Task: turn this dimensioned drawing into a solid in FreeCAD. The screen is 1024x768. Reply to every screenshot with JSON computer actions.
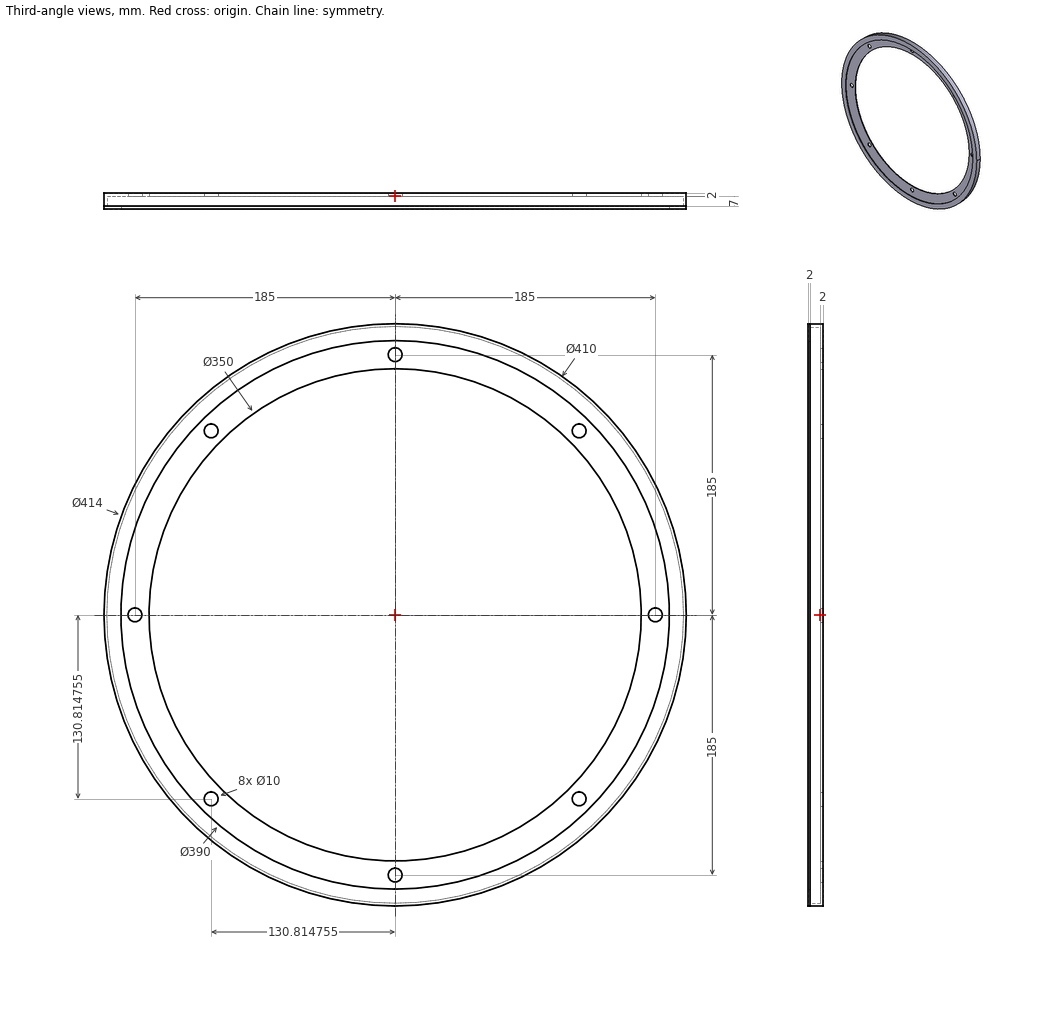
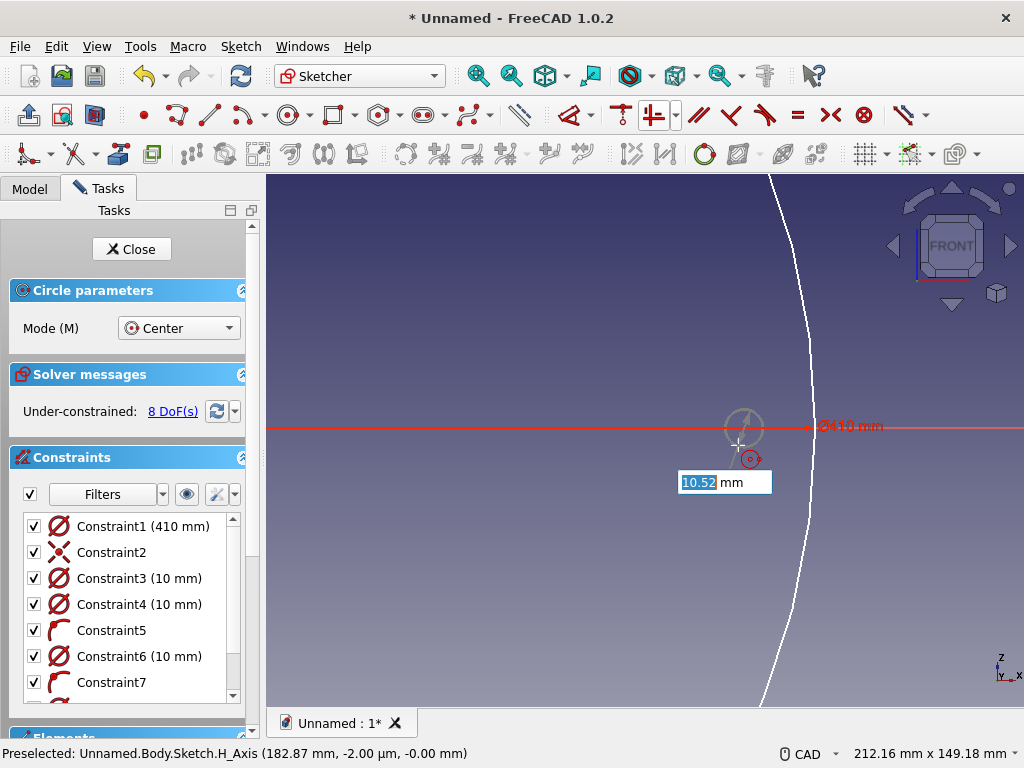
{"action": "type", "text": "10"}
{"action": "key", "text": "Return"}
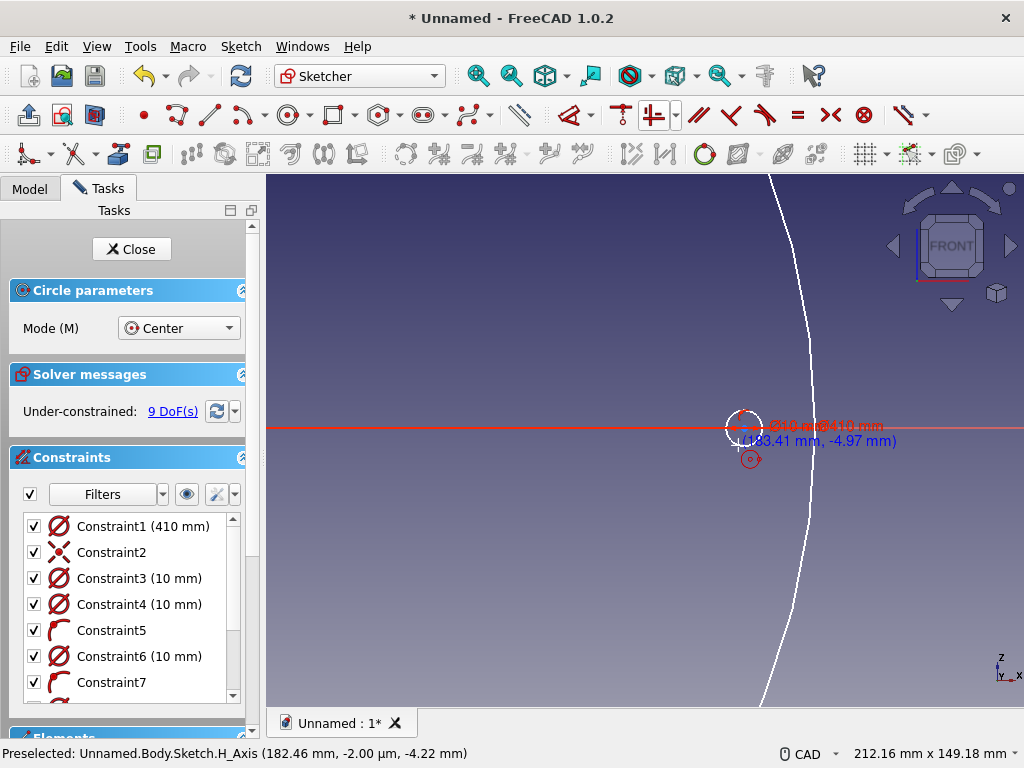
{"action": "scroll", "coordinate": [738, 445], "scroll_direction": "down", "scroll_amount": 7}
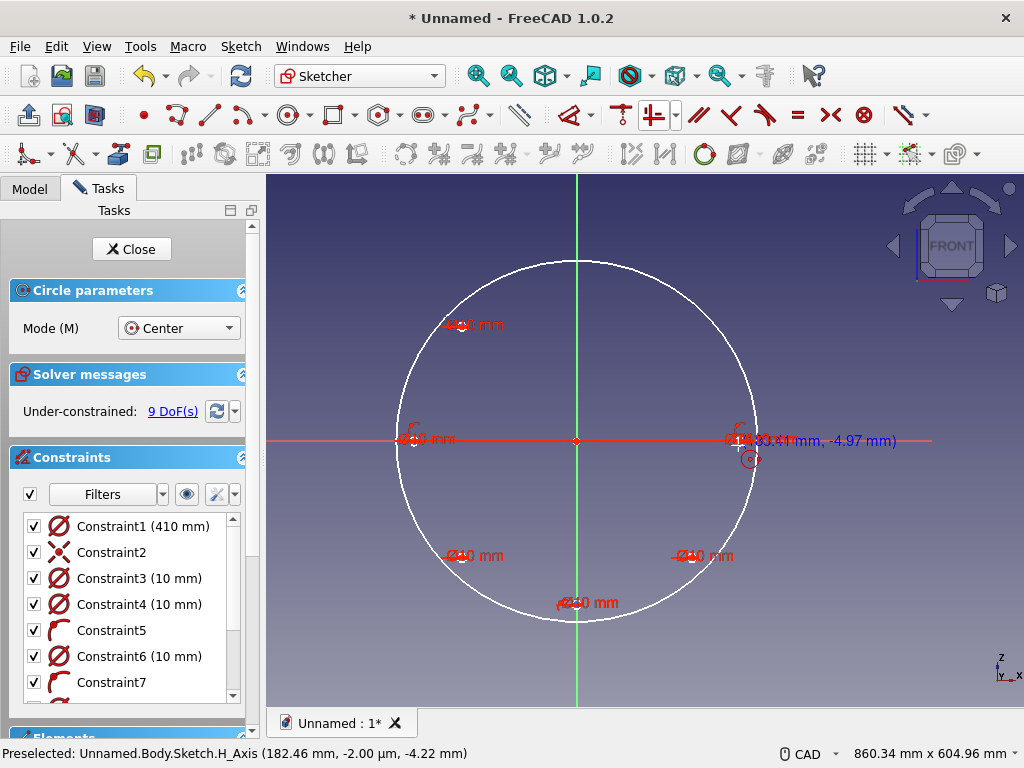
{"action": "left_click", "coordinate": [577, 441]}
{"action": "mouse_move", "coordinate": [686, 332]}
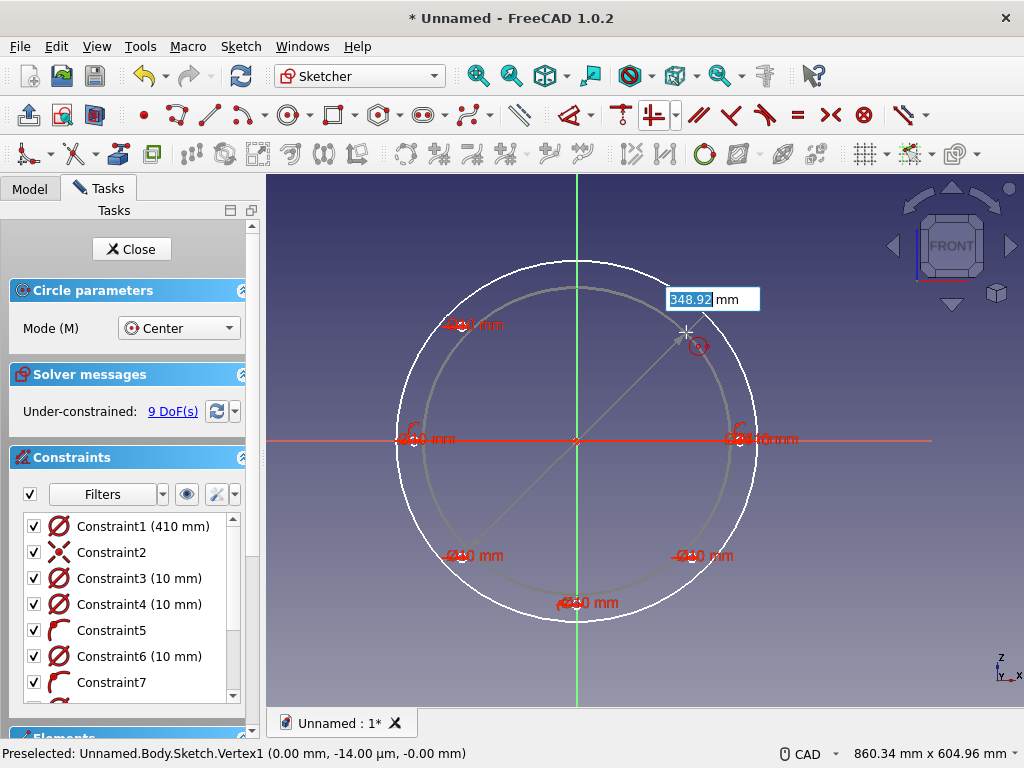
{"action": "type", "text": "350"}
{"action": "key", "text": "Return"}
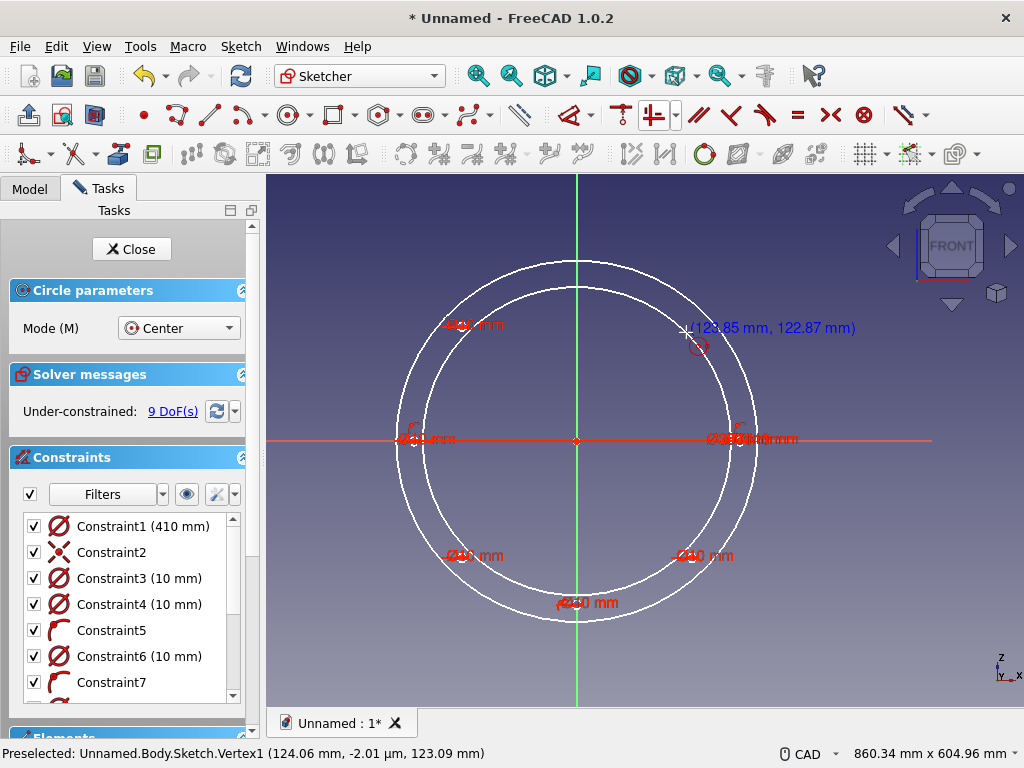
{"action": "scroll", "coordinate": [577, 278], "scroll_direction": "up", "scroll_amount": 9}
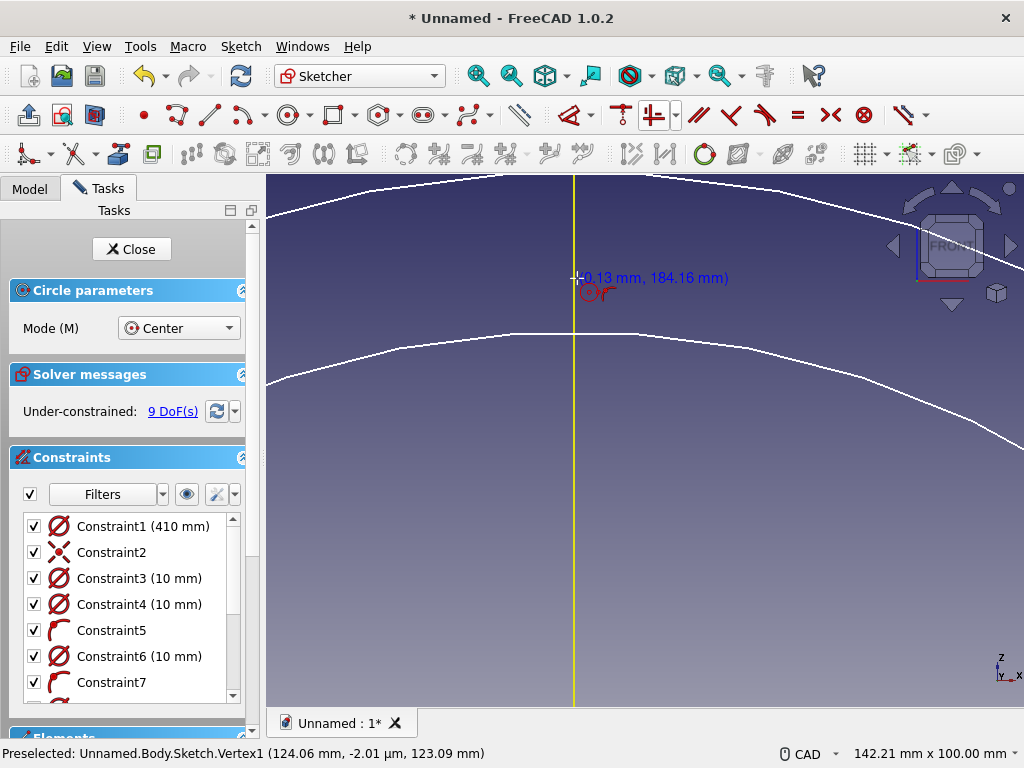
{"action": "scroll", "coordinate": [577, 277], "scroll_direction": "down", "scroll_amount": 9}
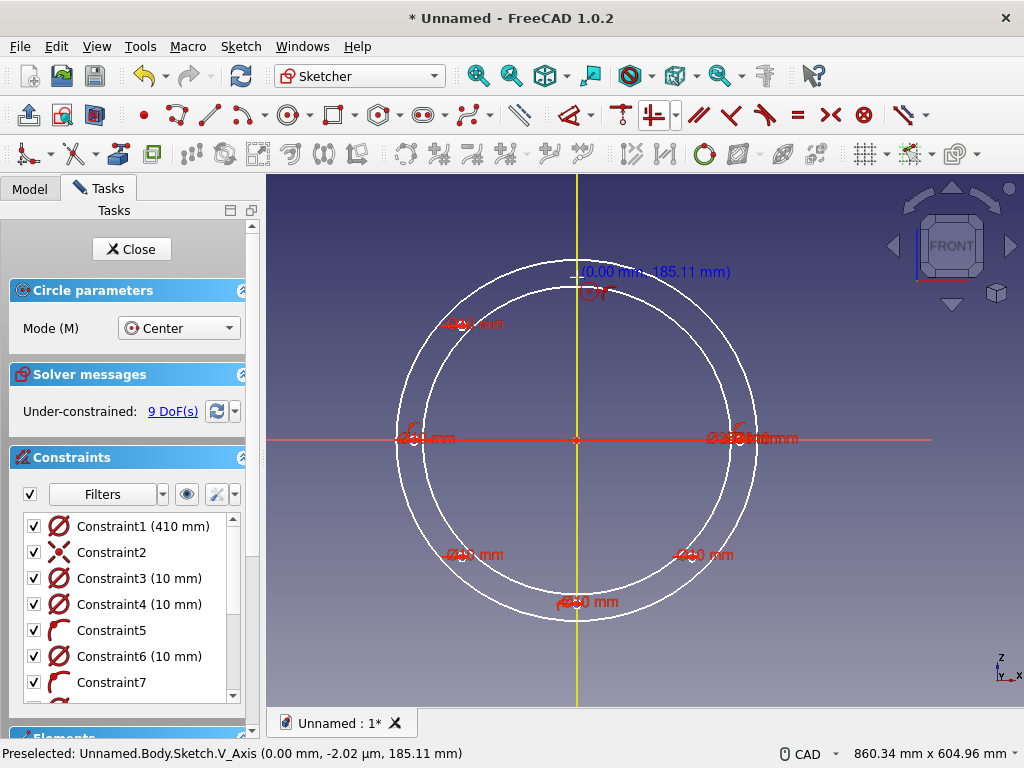
{"action": "scroll", "coordinate": [577, 277], "scroll_direction": "up", "scroll_amount": 3}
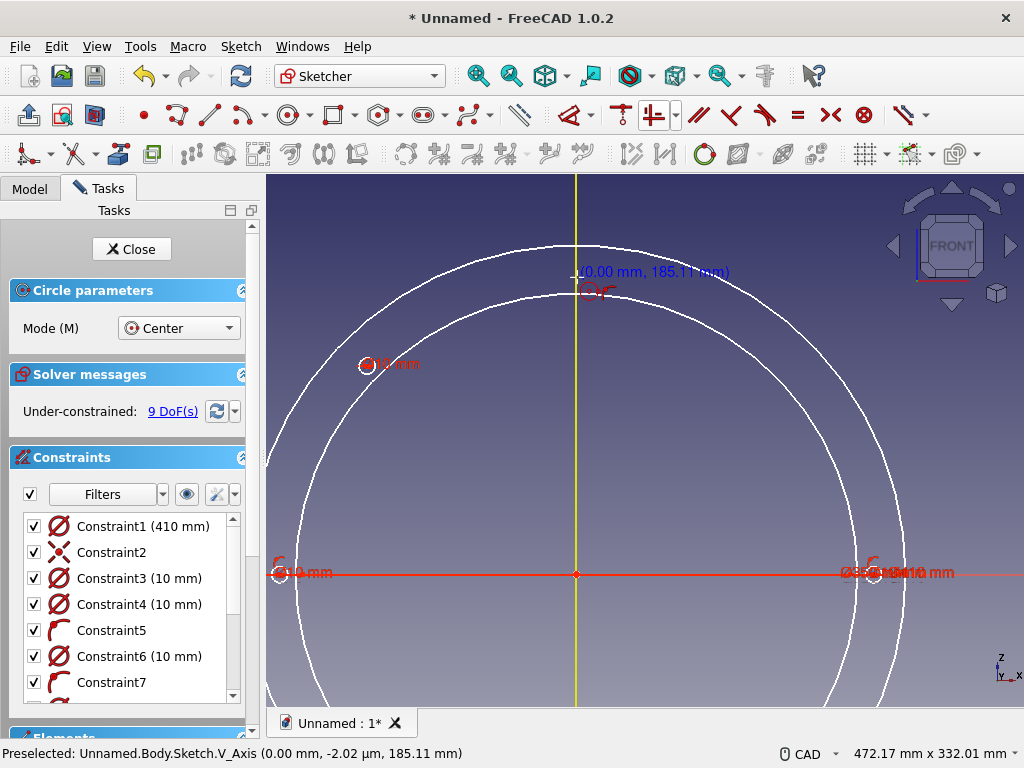
{"action": "left_click", "coordinate": [576, 278]}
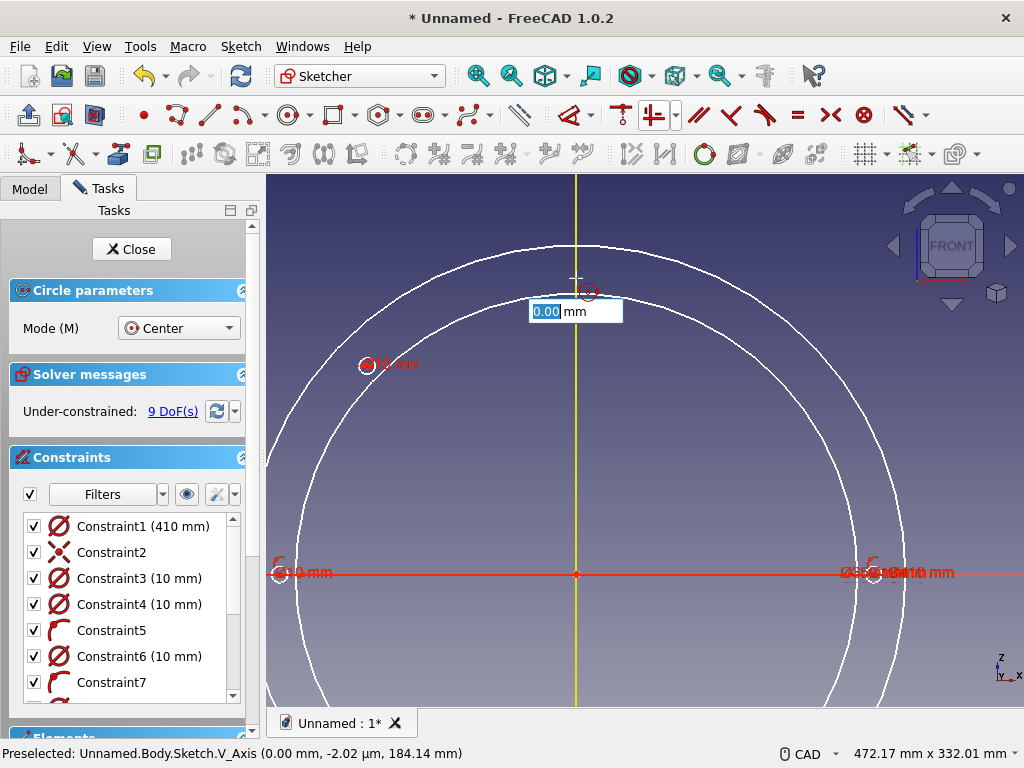
{"action": "scroll", "coordinate": [584, 275], "scroll_direction": "up", "scroll_amount": 4}
{"action": "mouse_move", "coordinate": [583, 274]}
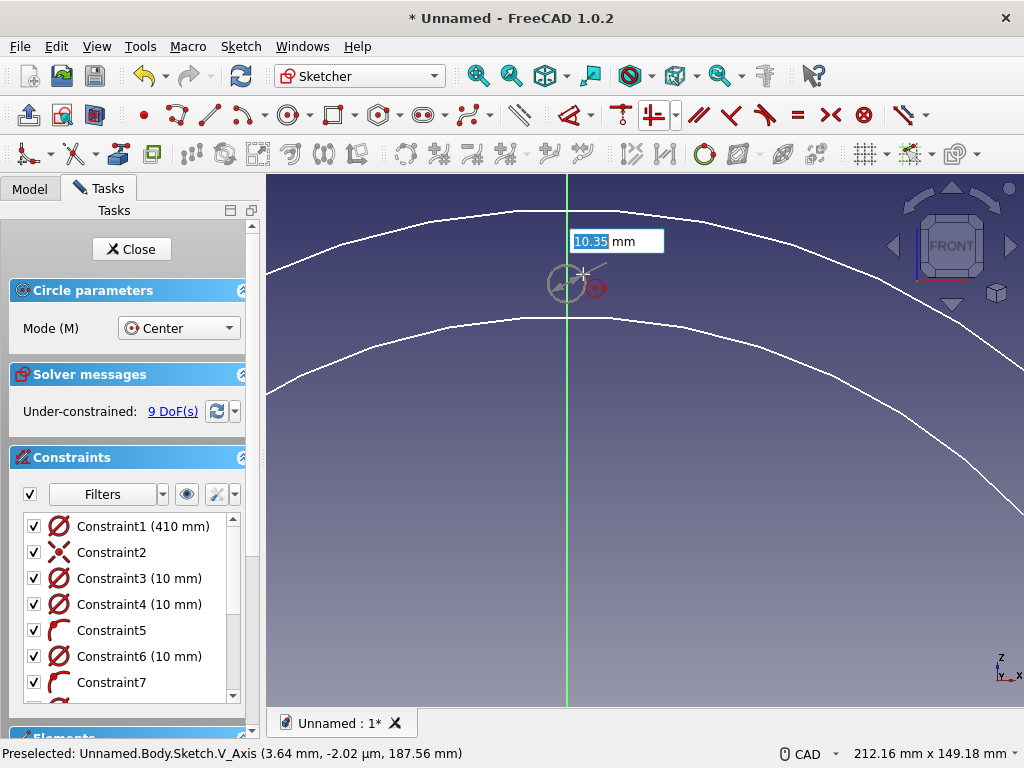
{"action": "type", "text": "10"}
{"action": "key", "text": "Return"}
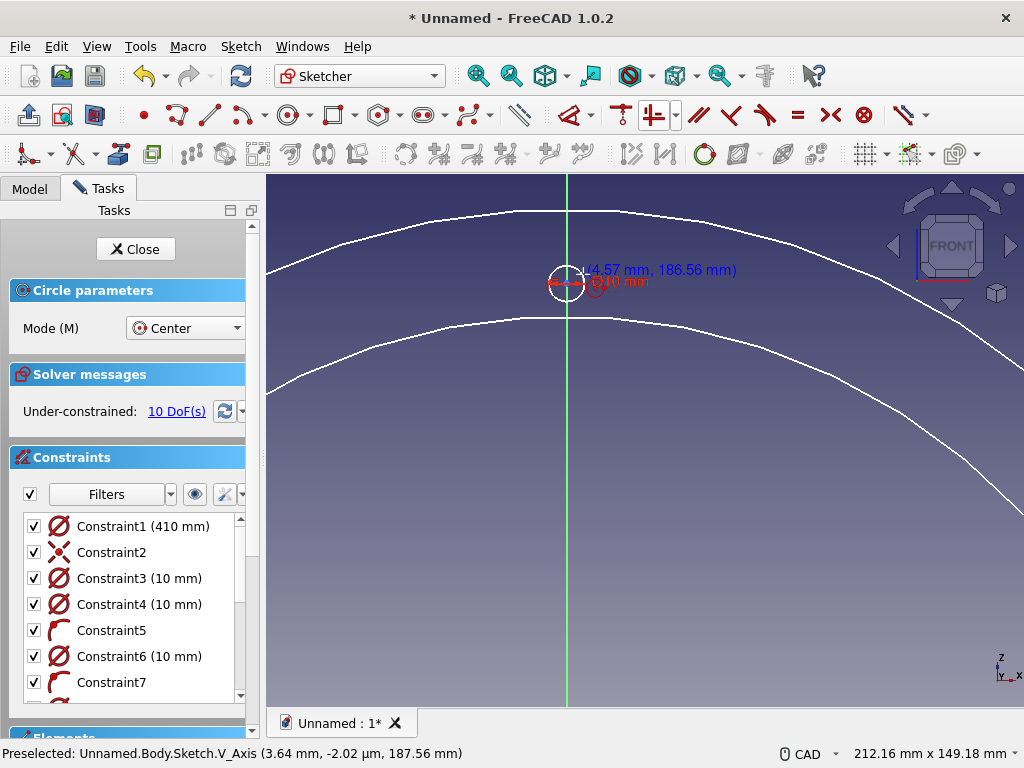
{"action": "scroll", "coordinate": [580, 276], "scroll_direction": "down", "scroll_amount": 7}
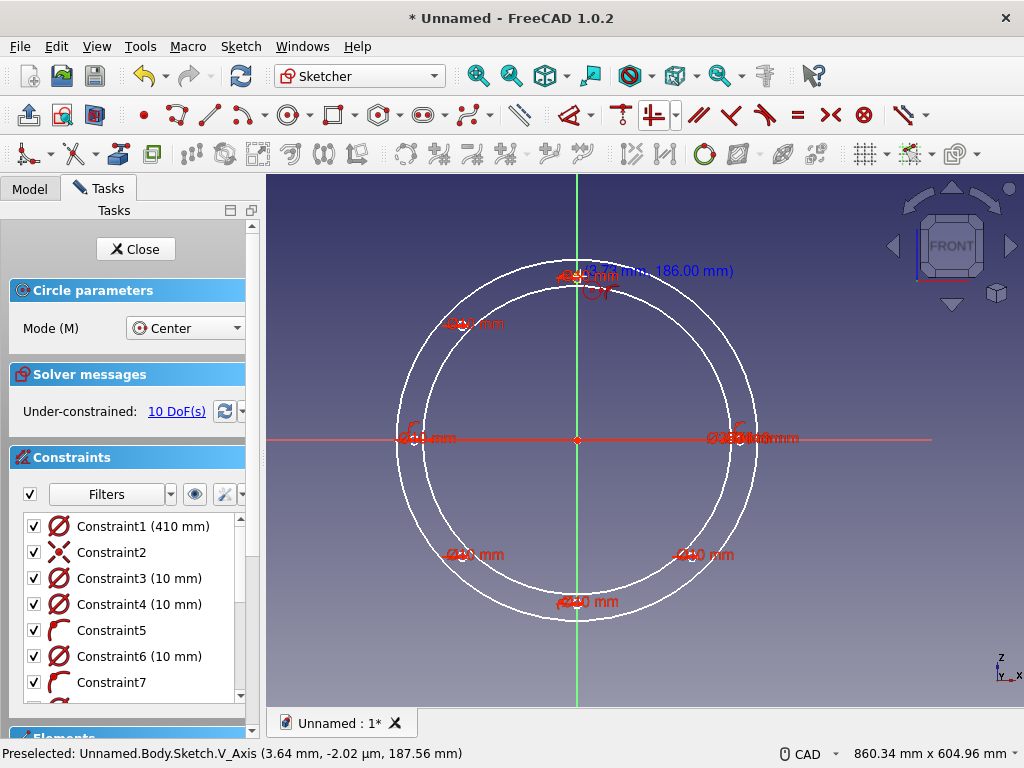
{"action": "scroll", "coordinate": [692, 325], "scroll_direction": "up", "scroll_amount": 9}